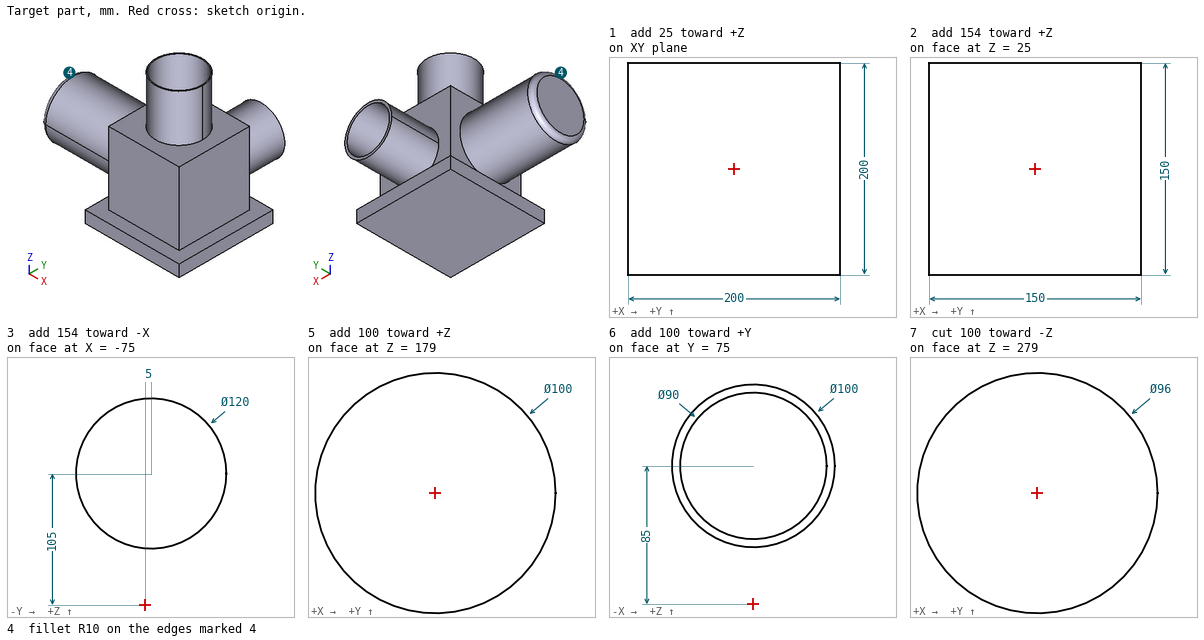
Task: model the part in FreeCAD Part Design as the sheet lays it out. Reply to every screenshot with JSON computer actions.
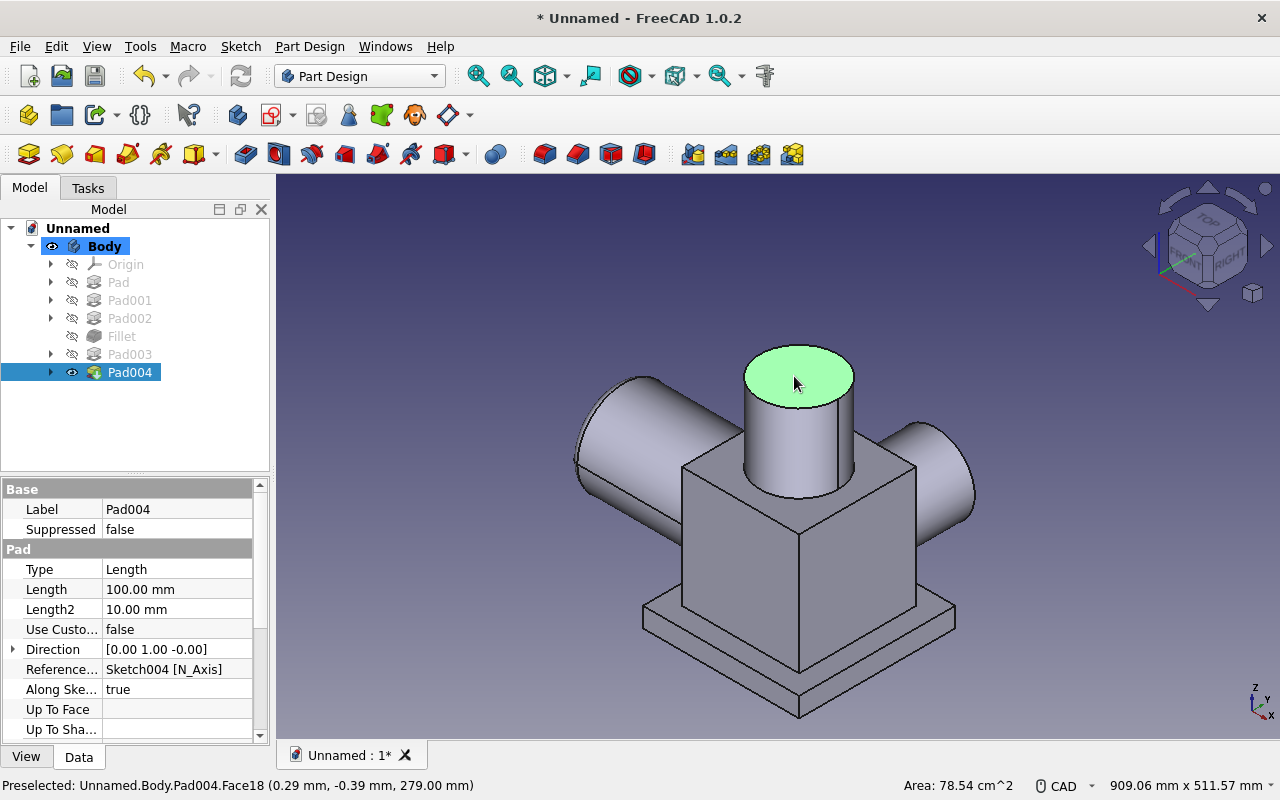
{"action": "left_click", "coordinate": [270, 116]}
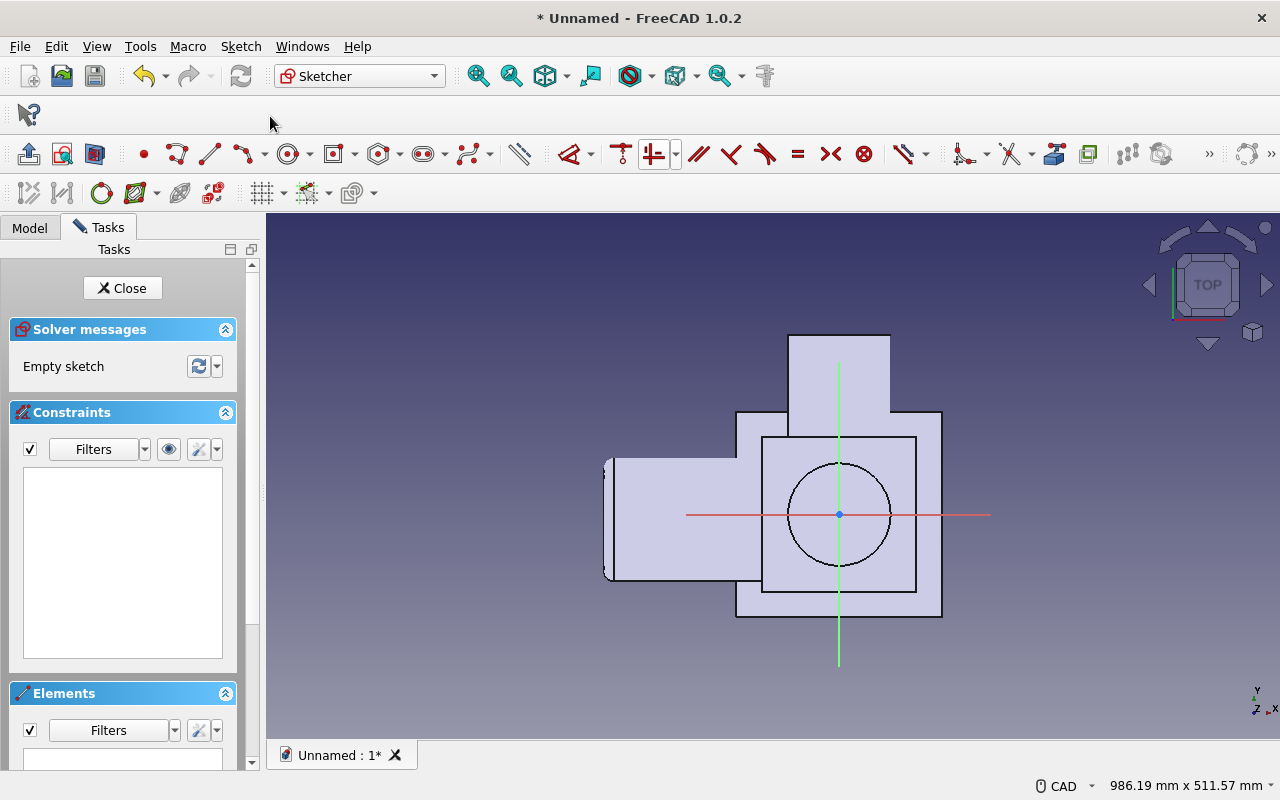
{"action": "scroll", "coordinate": [897, 531], "scroll_direction": "up", "scroll_amount": 6}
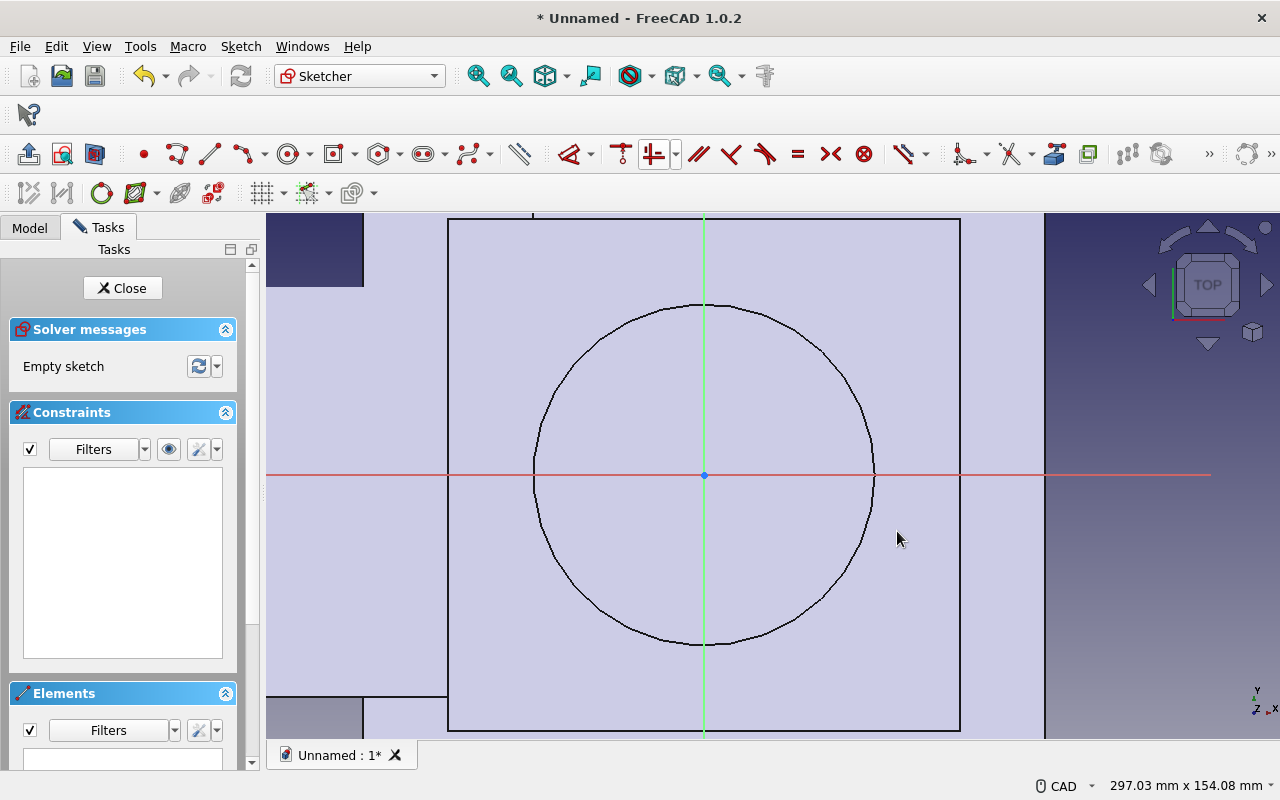
{"action": "key", "text": "g c"}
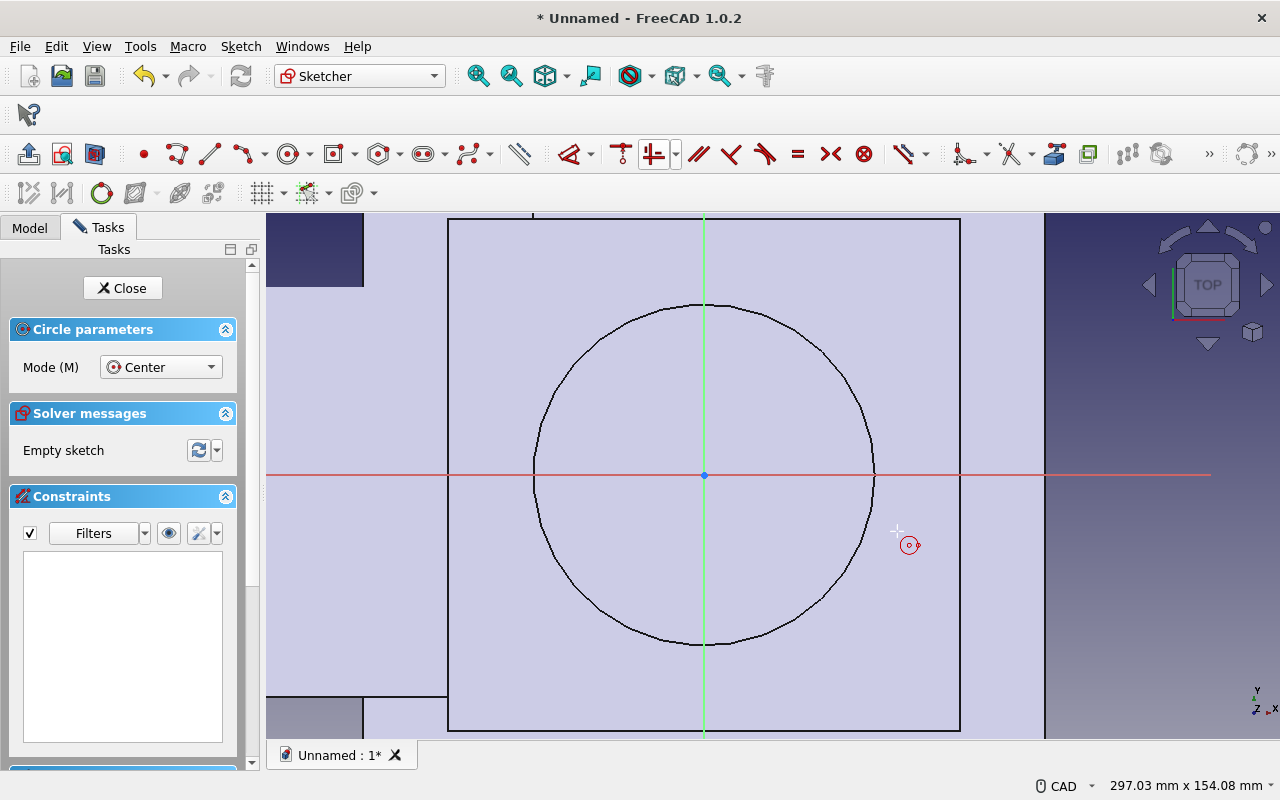
{"action": "left_click", "coordinate": [704, 475]}
{"action": "mouse_move", "coordinate": [820, 359]}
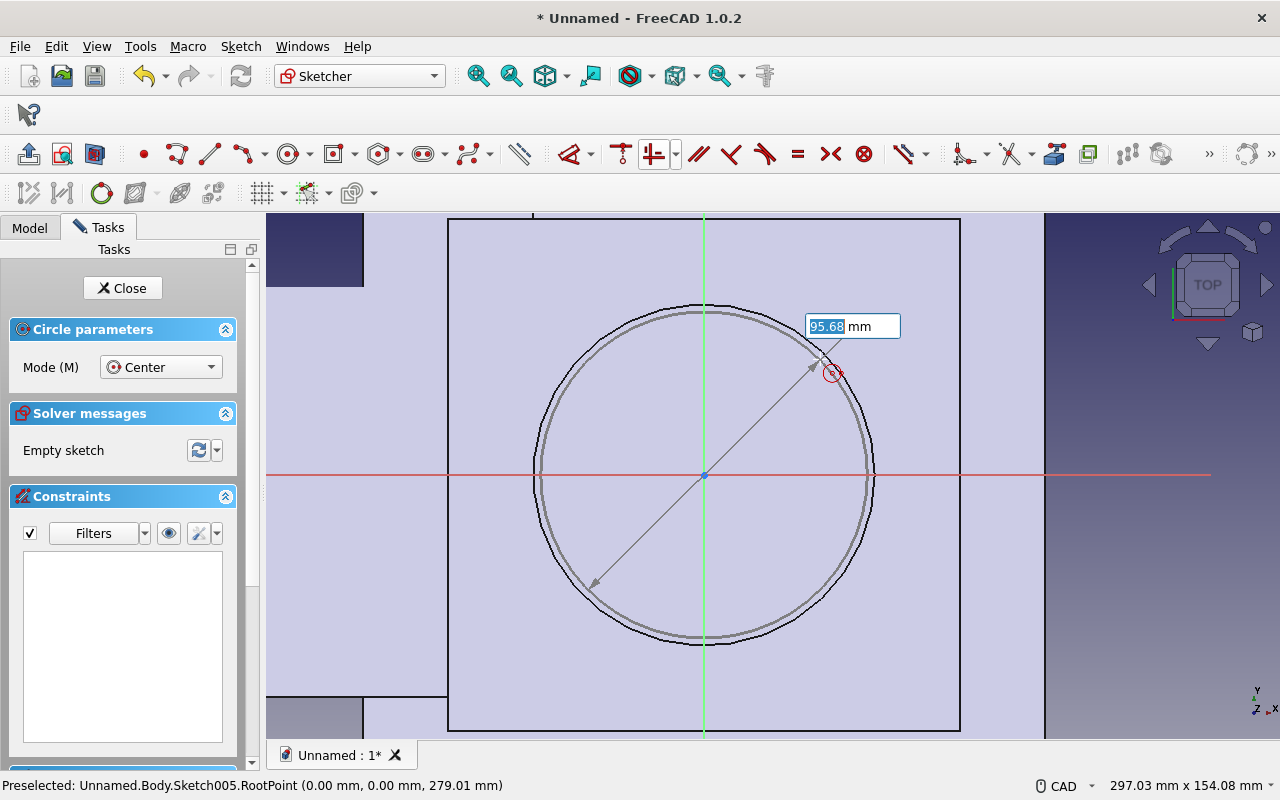
{"action": "type", "text": "96"}
{"action": "key", "text": "Return"}
{"action": "key", "text": "Escape"}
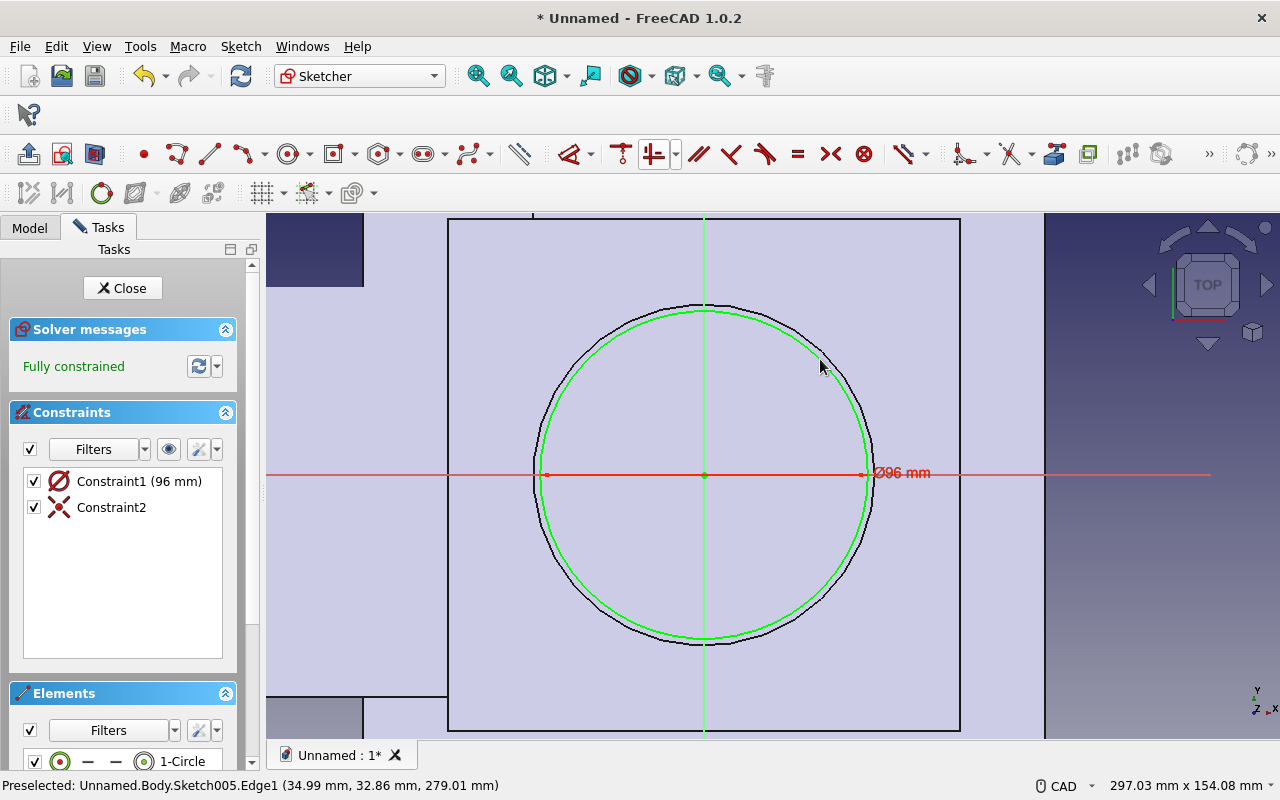
{"action": "left_click", "coordinate": [123, 288]}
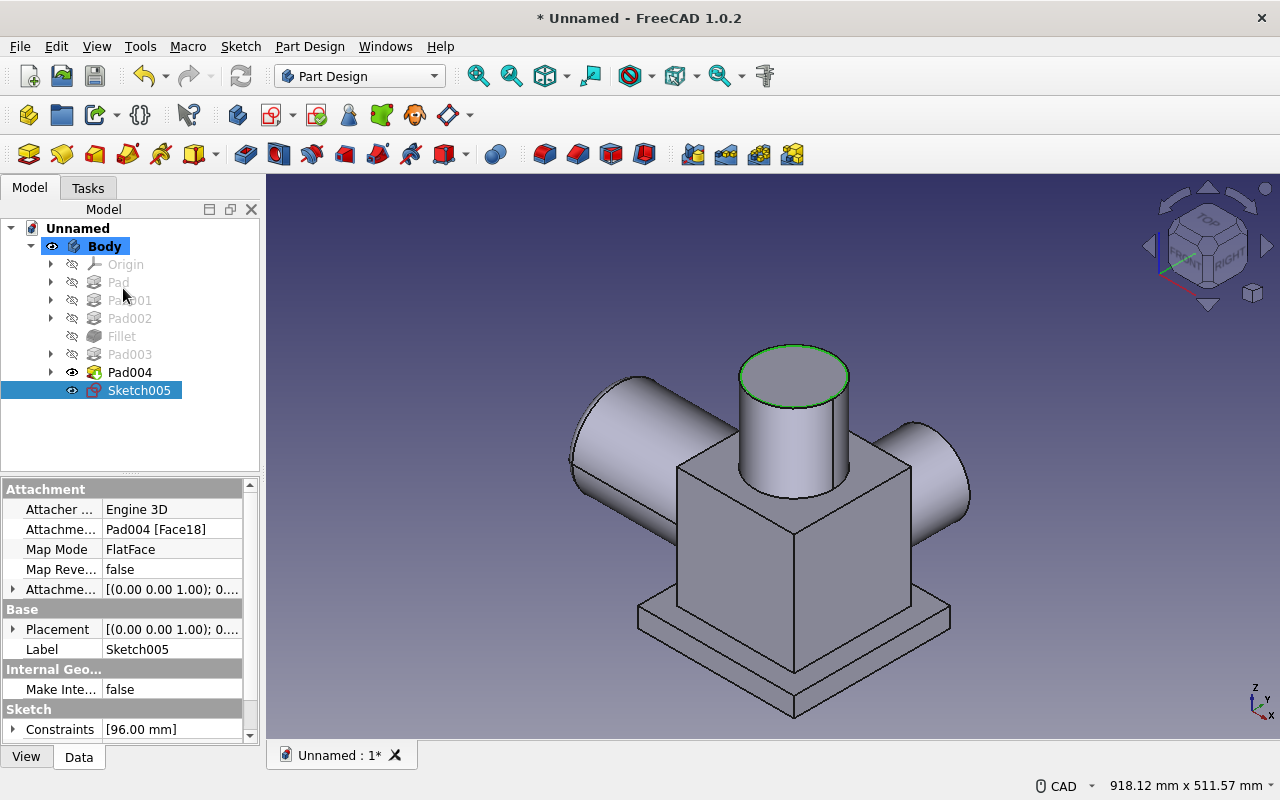
{"action": "left_click", "coordinate": [246, 154]}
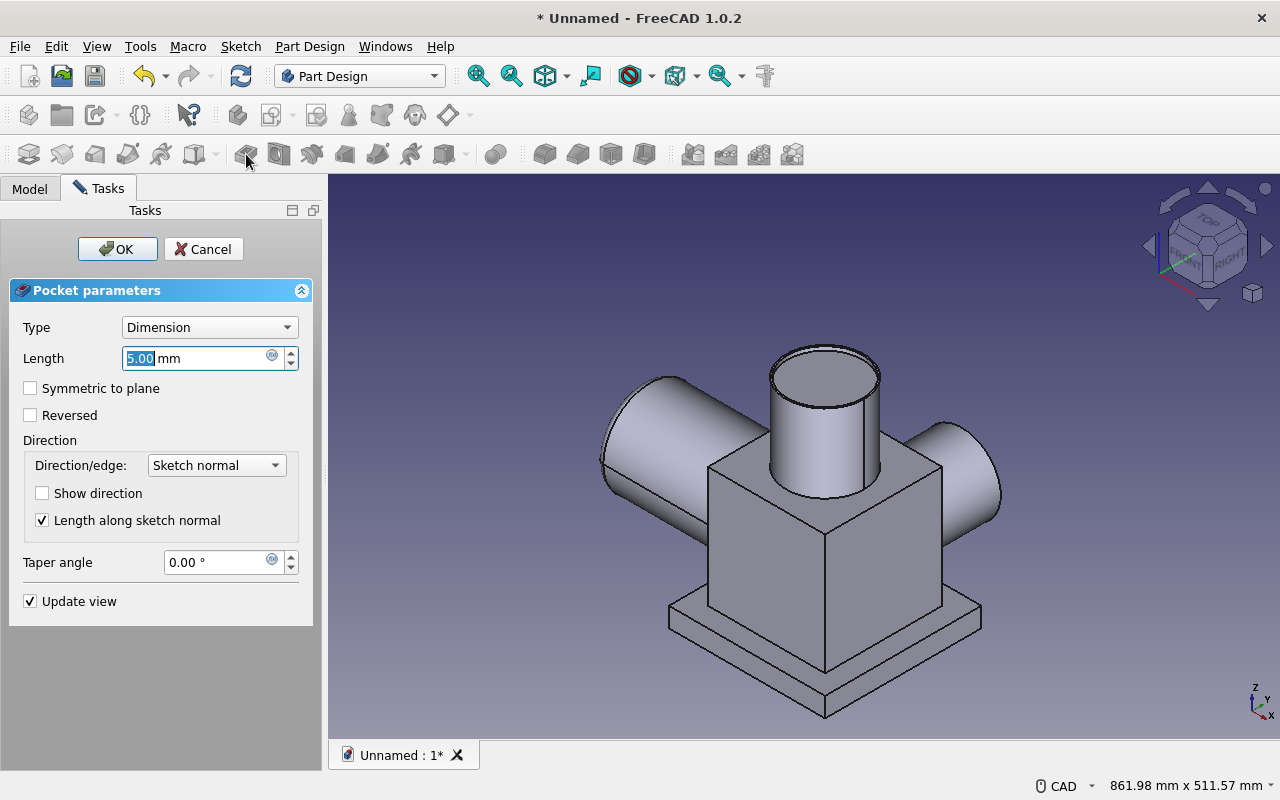
{"action": "type", "text": "100"}
{"action": "key", "text": "Tab"}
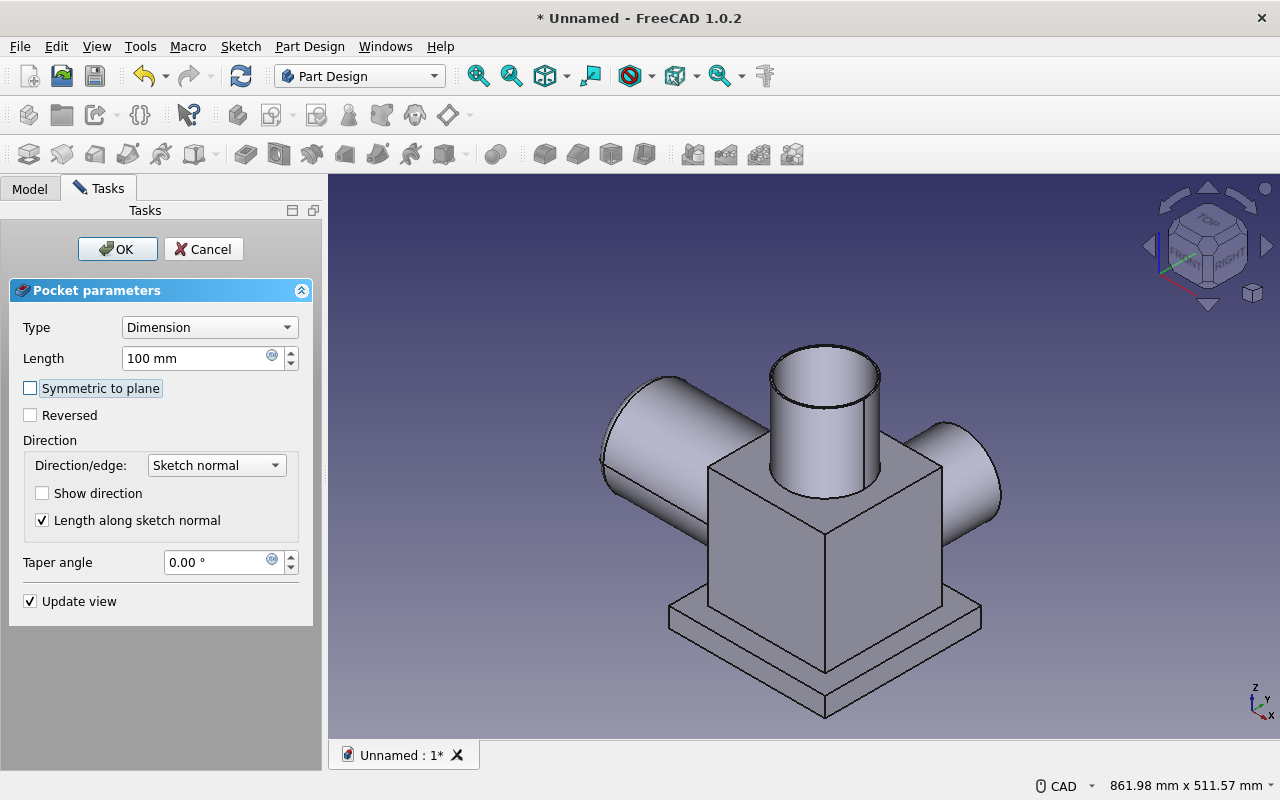
{"action": "left_click", "coordinate": [118, 249]}